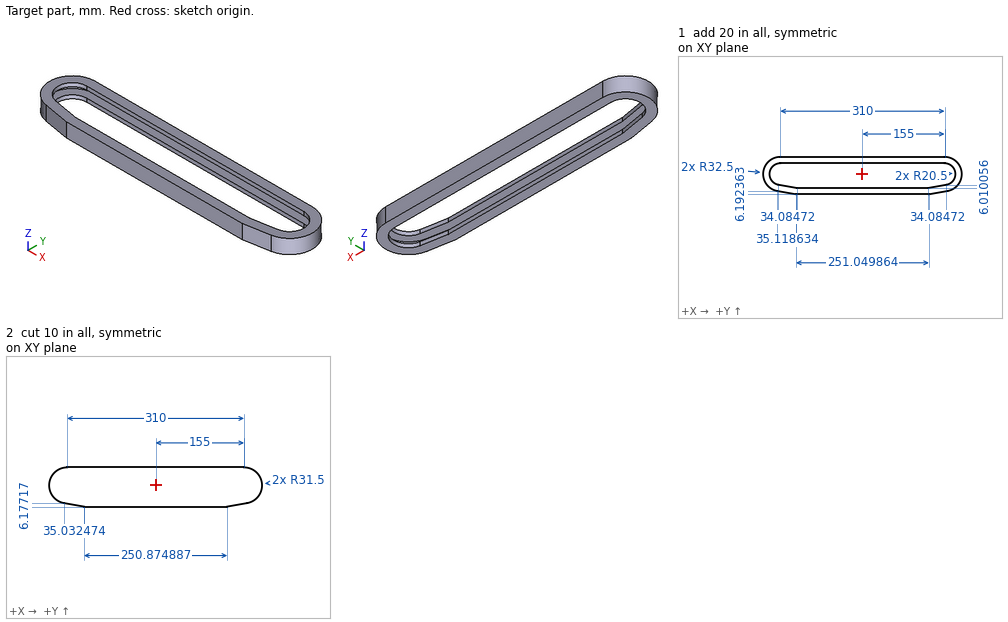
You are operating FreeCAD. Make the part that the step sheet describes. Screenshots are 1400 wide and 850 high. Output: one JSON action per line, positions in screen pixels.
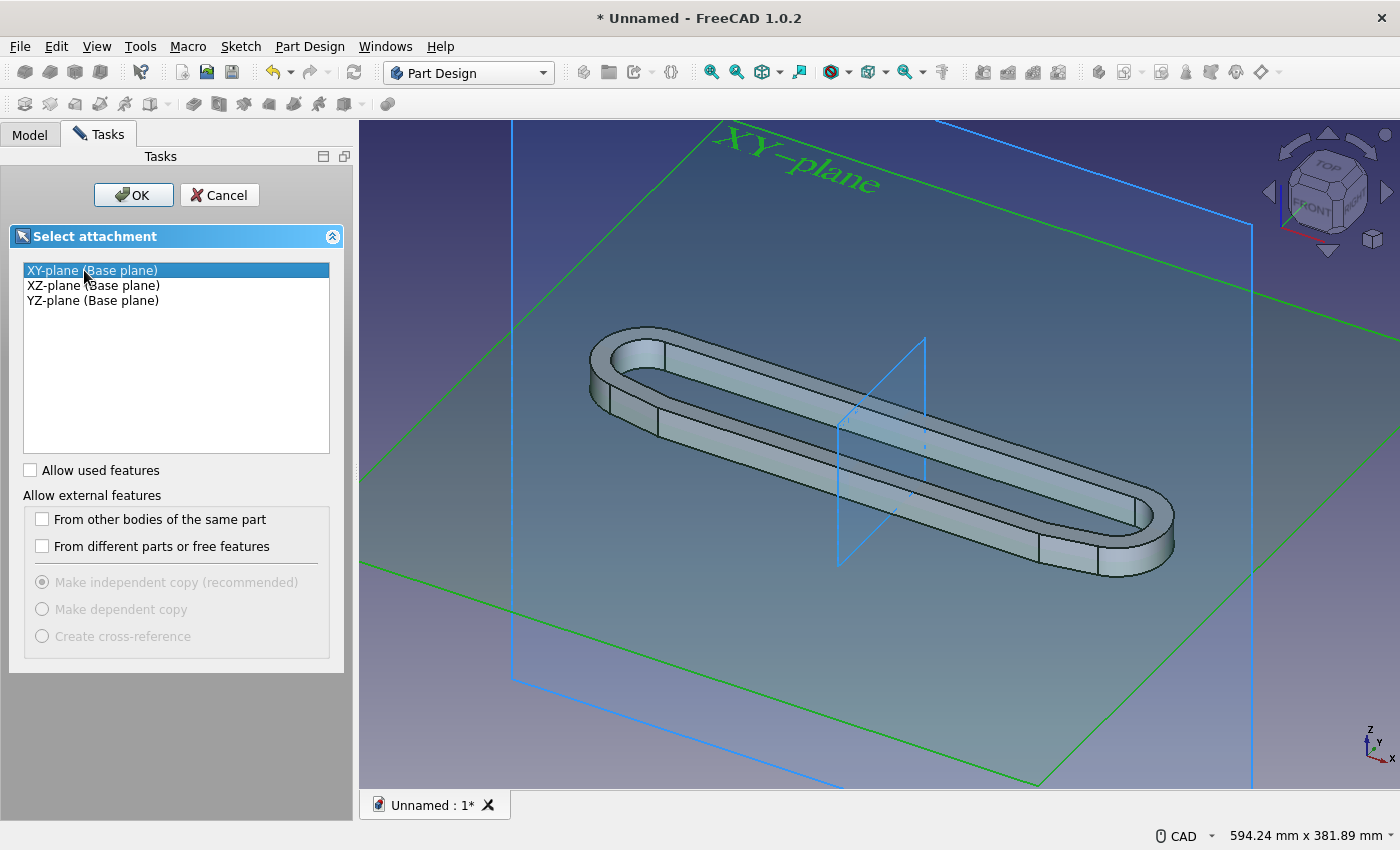
{"action": "left_click", "coordinate": [134, 195]}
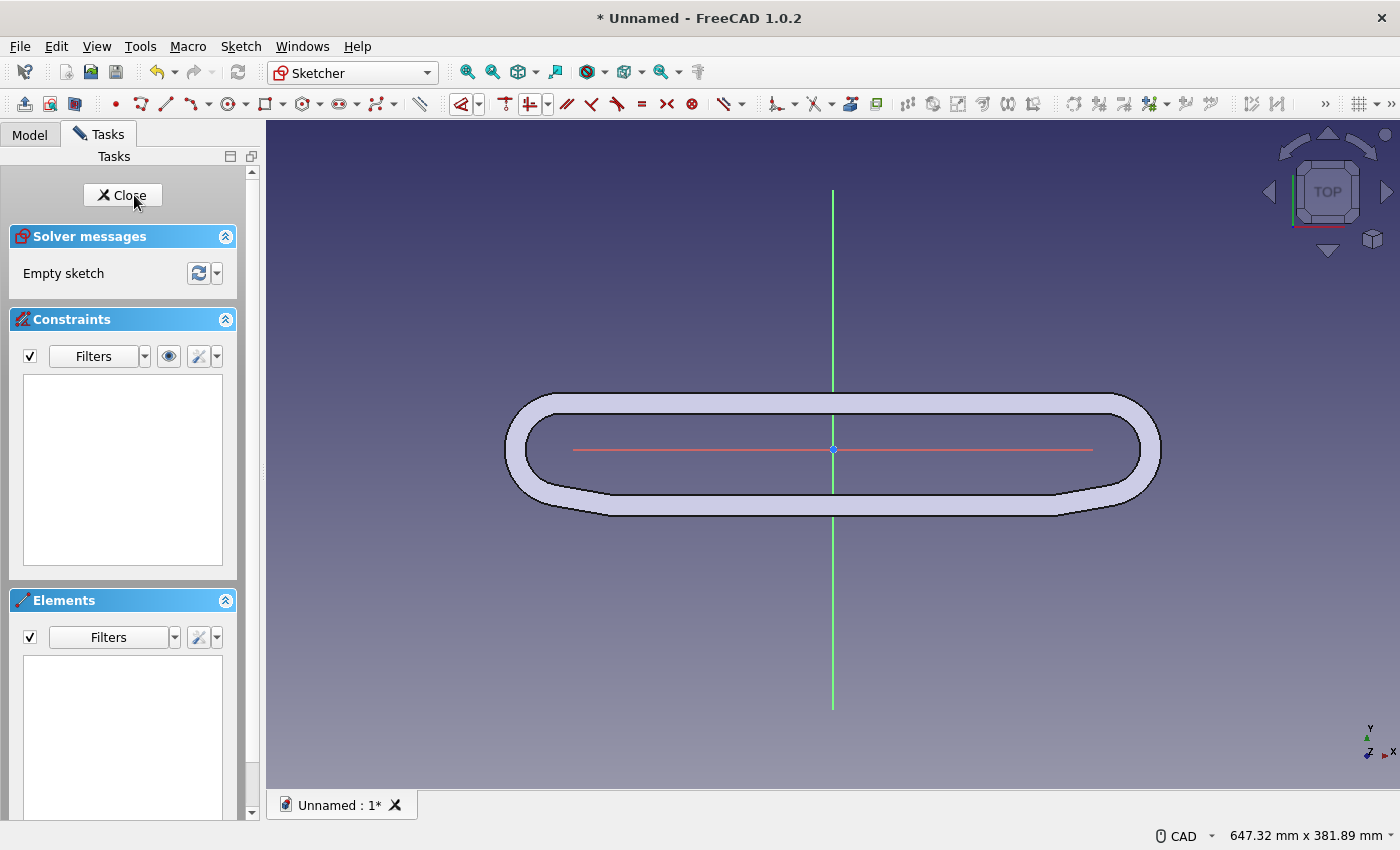
{"action": "key", "text": "q s"}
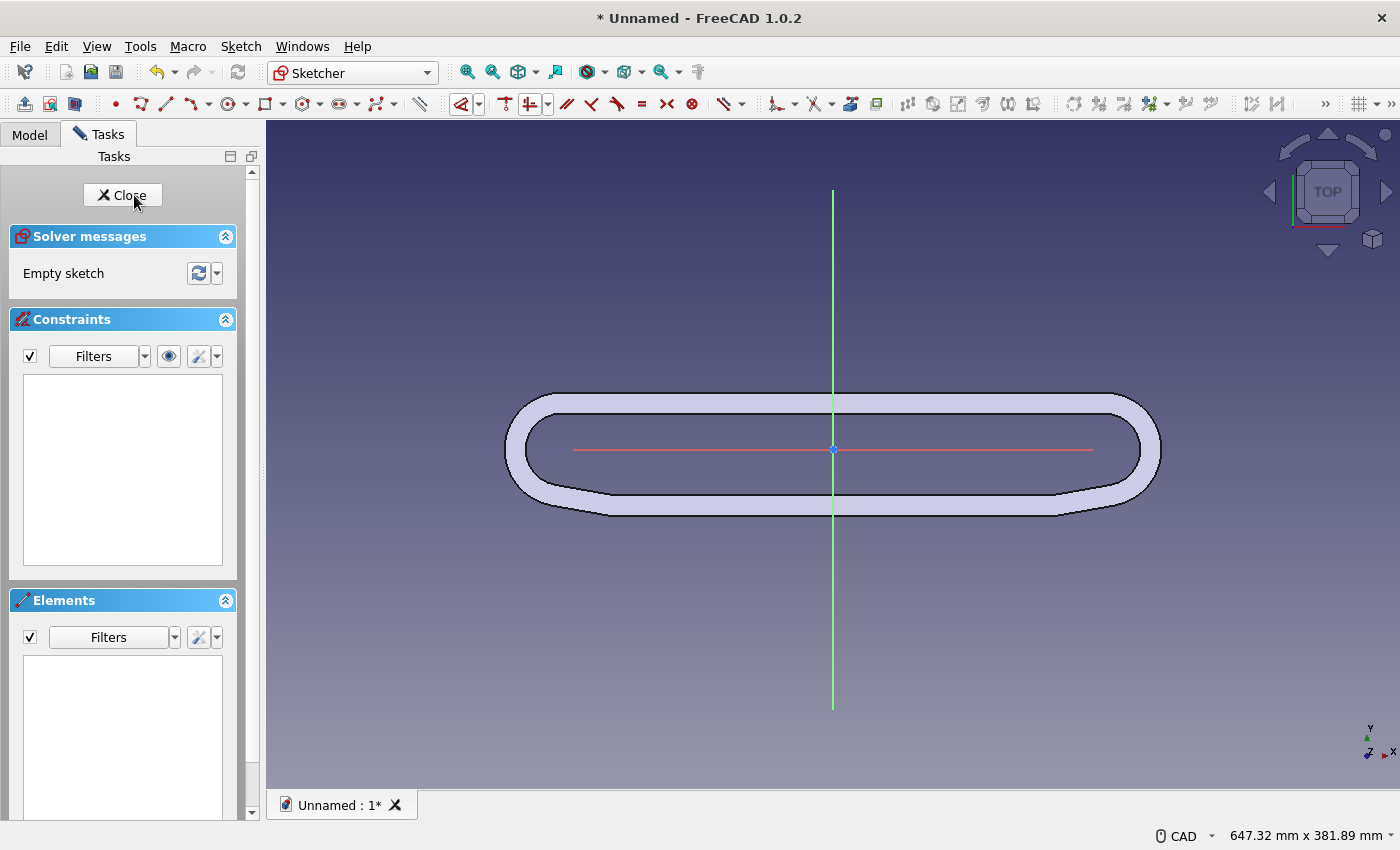
{"action": "left_click", "coordinate": [166, 104]}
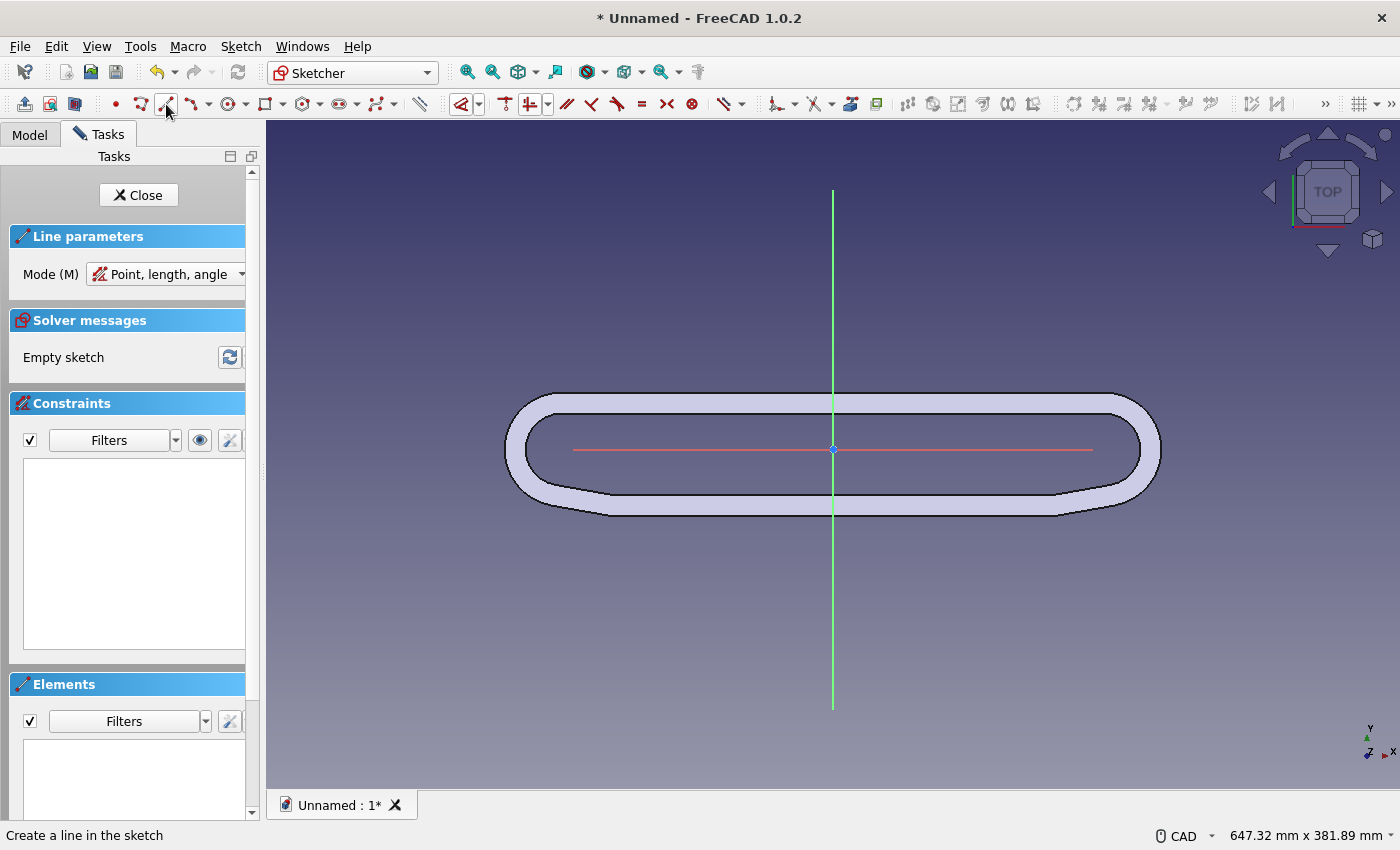
{"action": "left_click", "coordinate": [1105, 394]}
{"action": "left_click", "coordinate": [561, 394]}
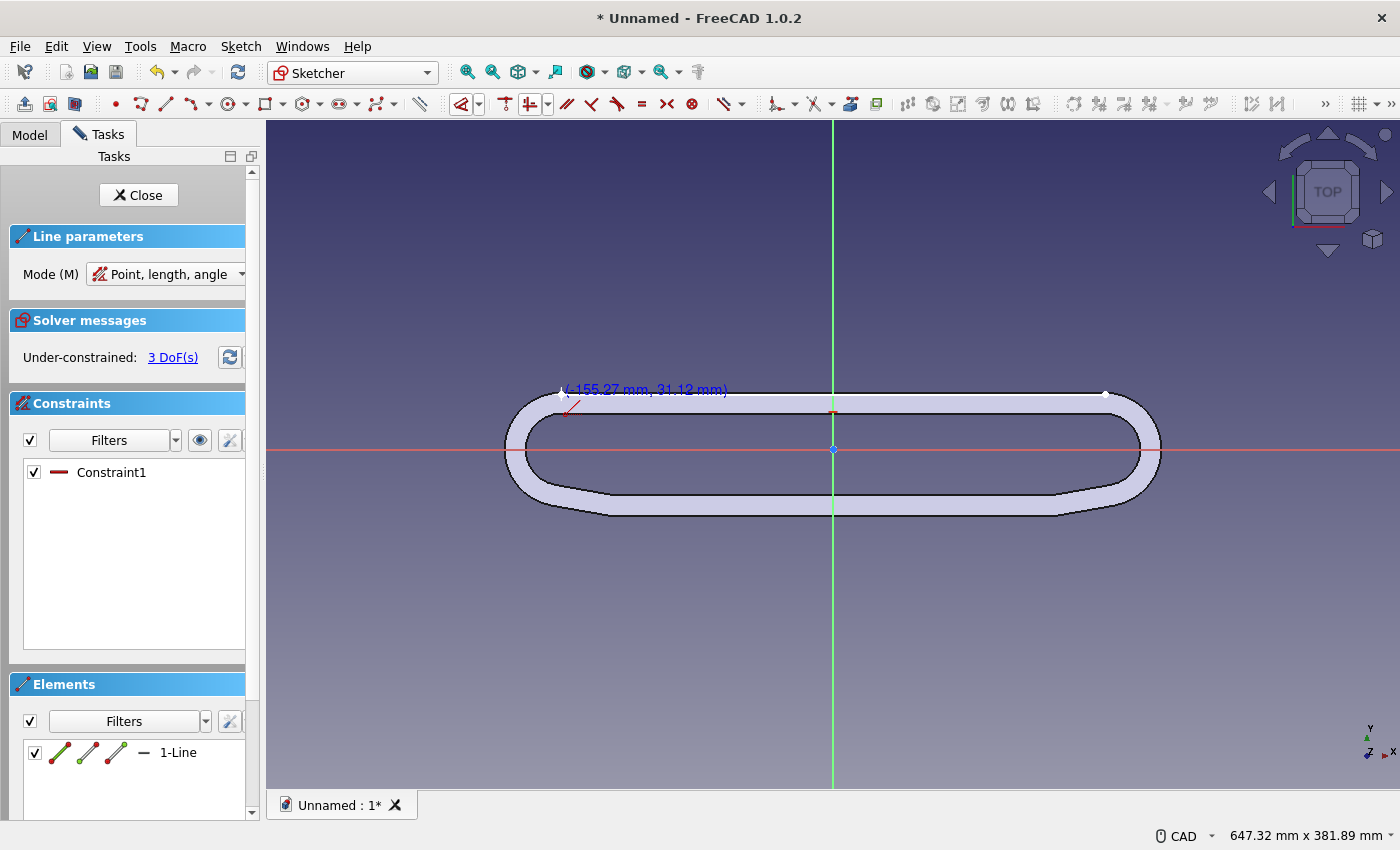
{"action": "left_click", "coordinate": [141, 104]}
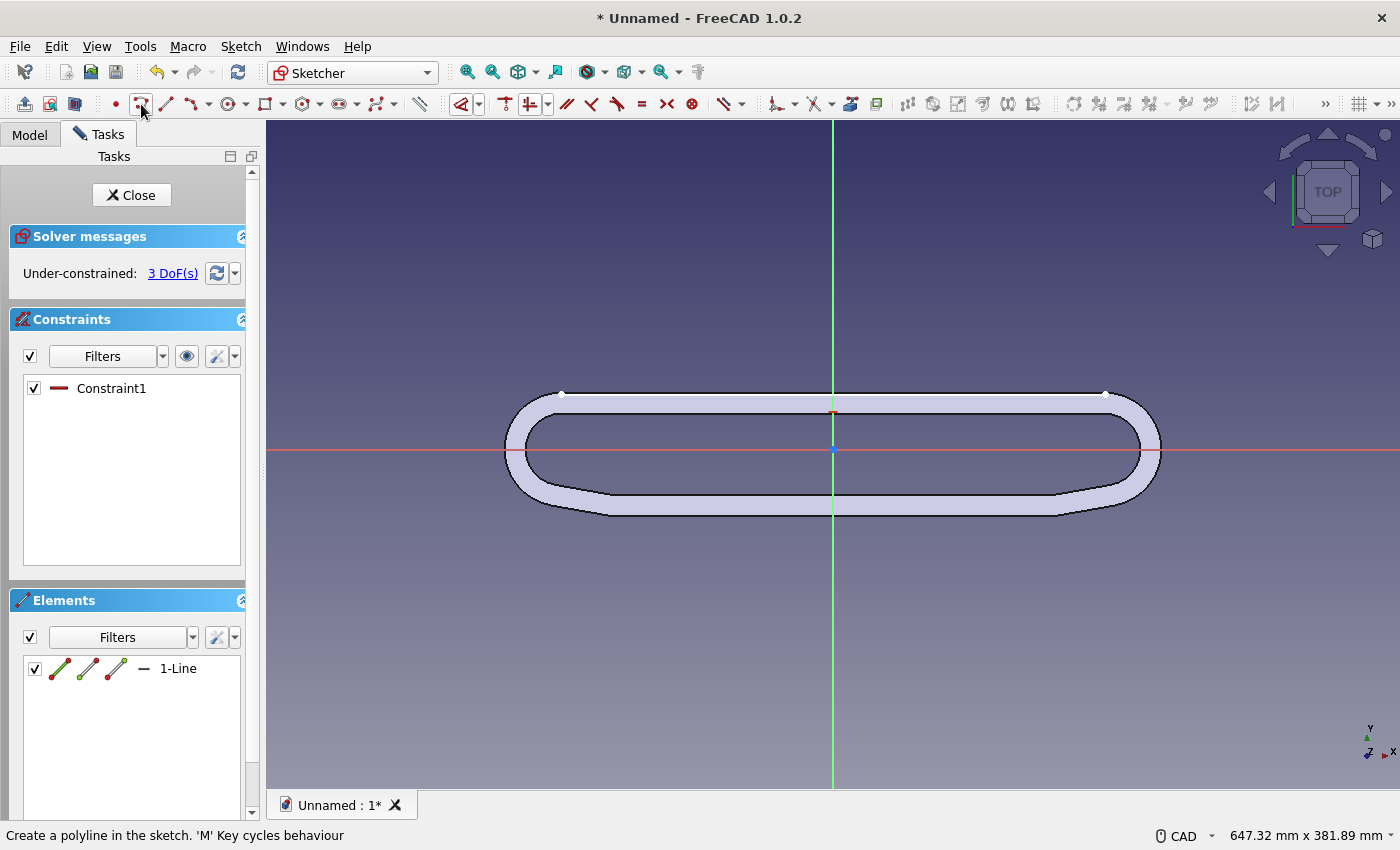
{"action": "left_click", "coordinate": [552, 504]}
{"action": "left_click", "coordinate": [613, 515]}
{"action": "left_click", "coordinate": [1053, 515]}
{"action": "left_click", "coordinate": [1114, 504]}
{"action": "right_click", "coordinate": [1114, 504]}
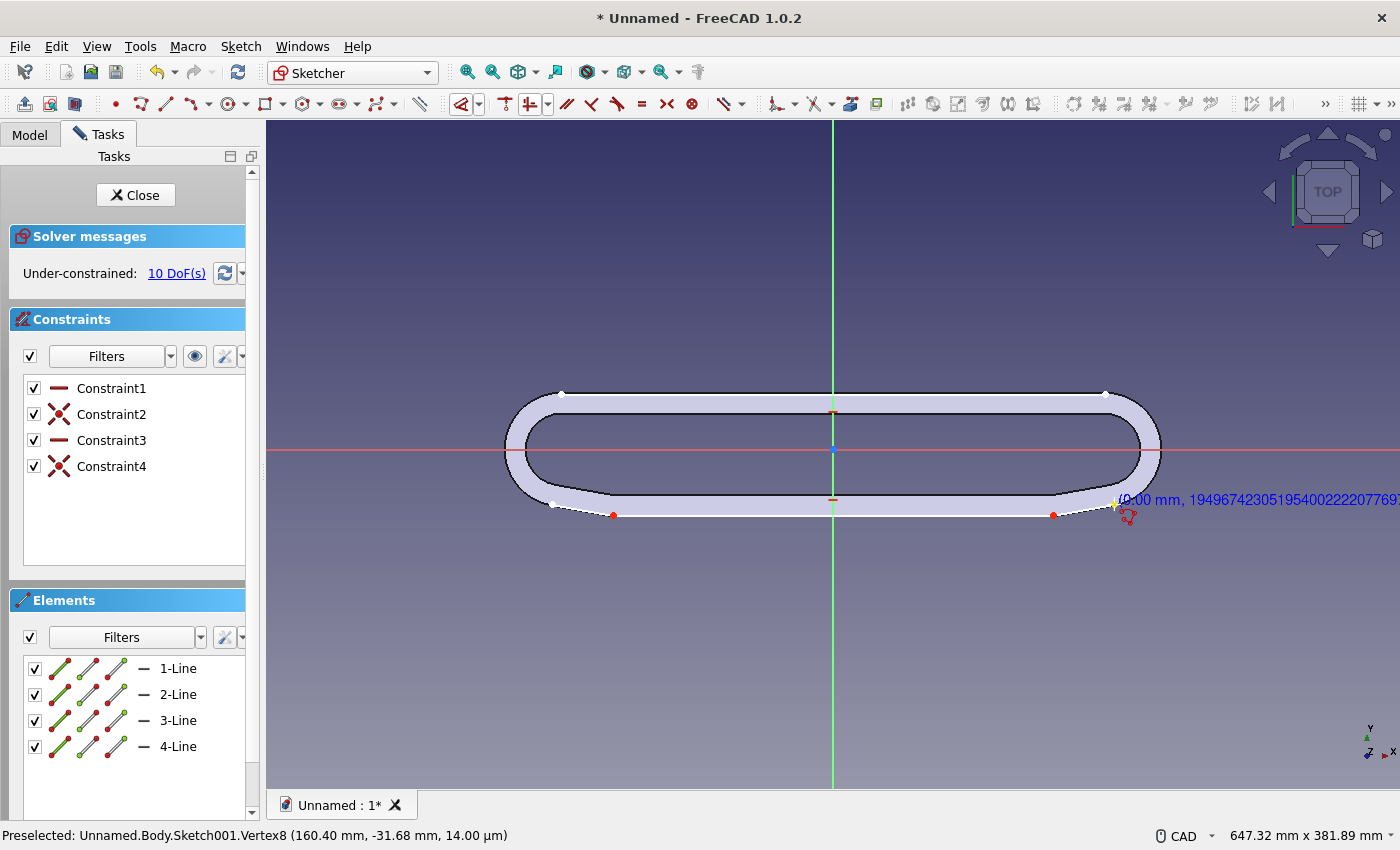
{"action": "key", "text": "g 3 a"}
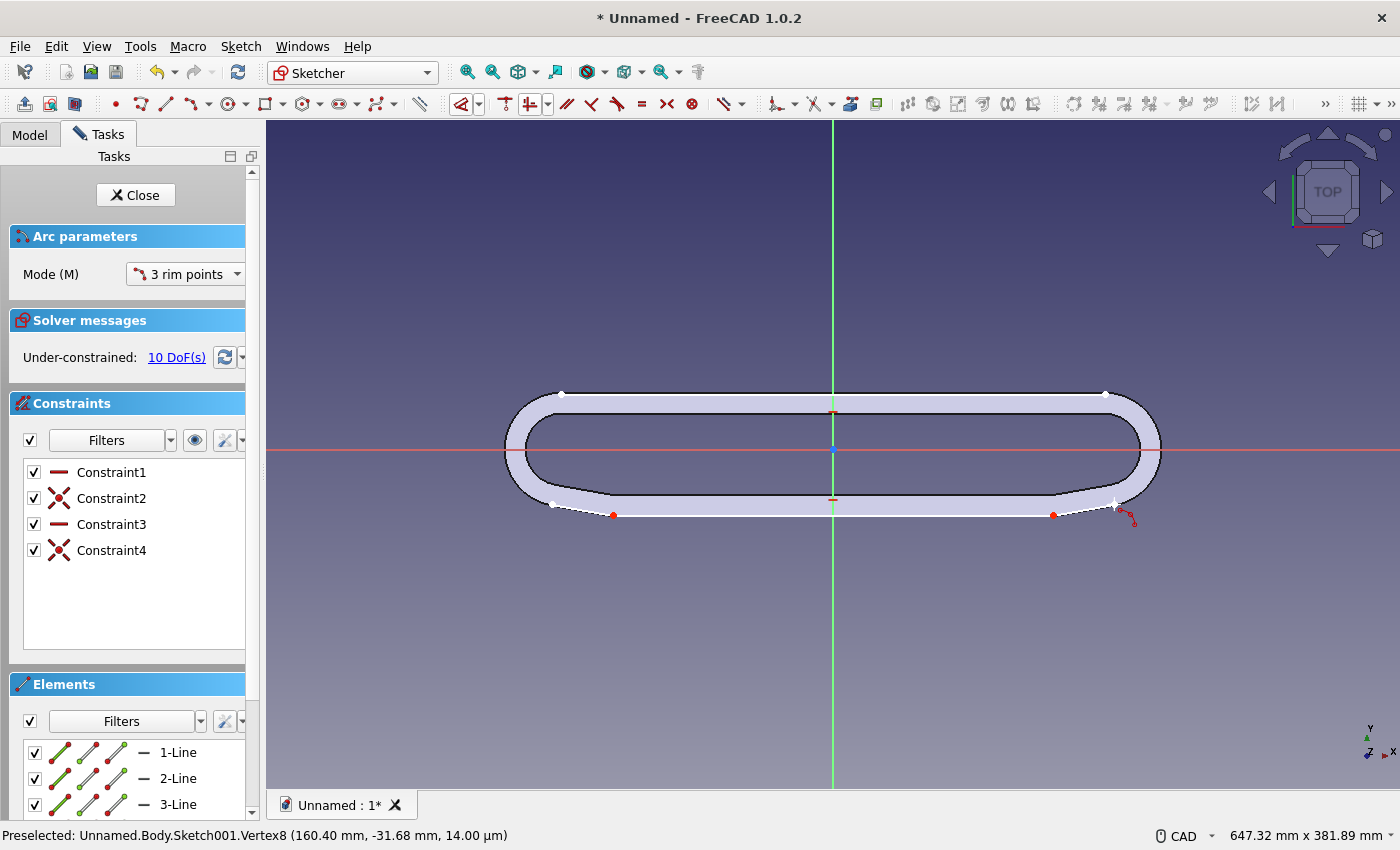
{"action": "left_click", "coordinate": [561, 395]}
{"action": "left_click", "coordinate": [552, 505]}
{"action": "left_click", "coordinate": [510, 429]}